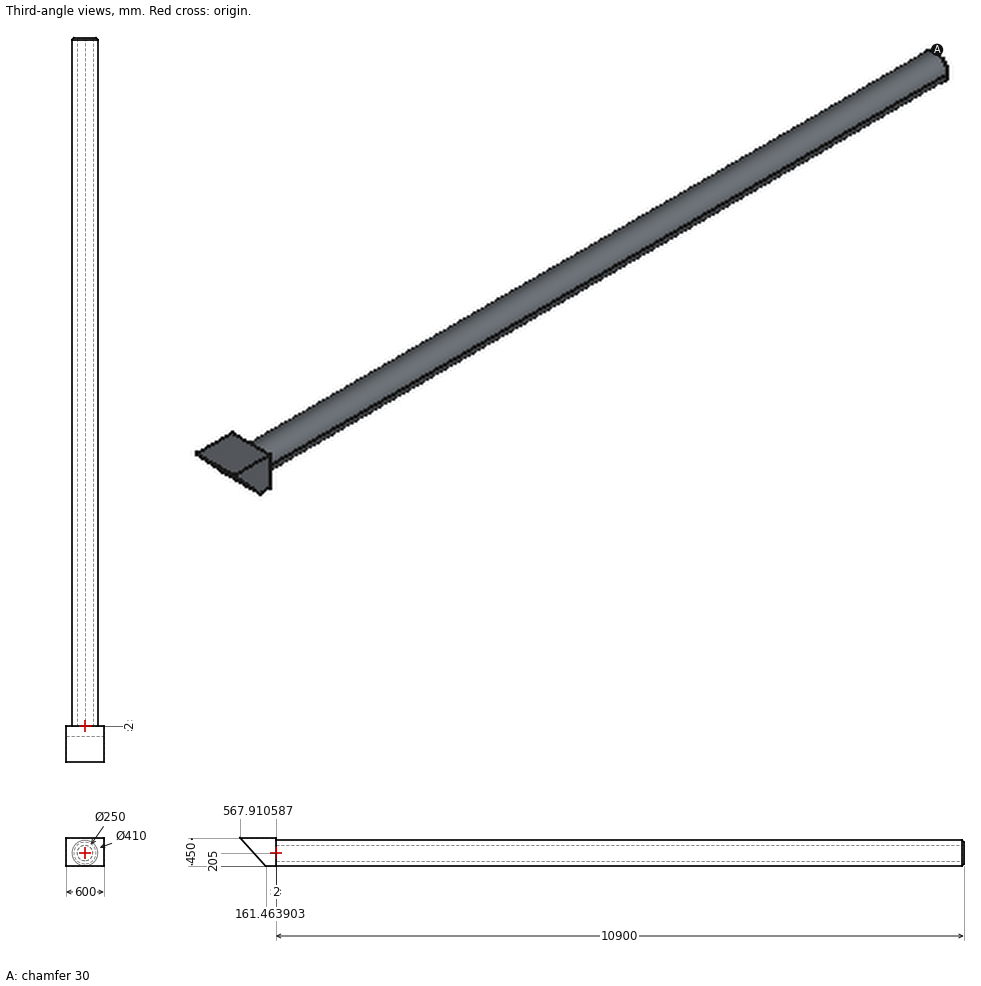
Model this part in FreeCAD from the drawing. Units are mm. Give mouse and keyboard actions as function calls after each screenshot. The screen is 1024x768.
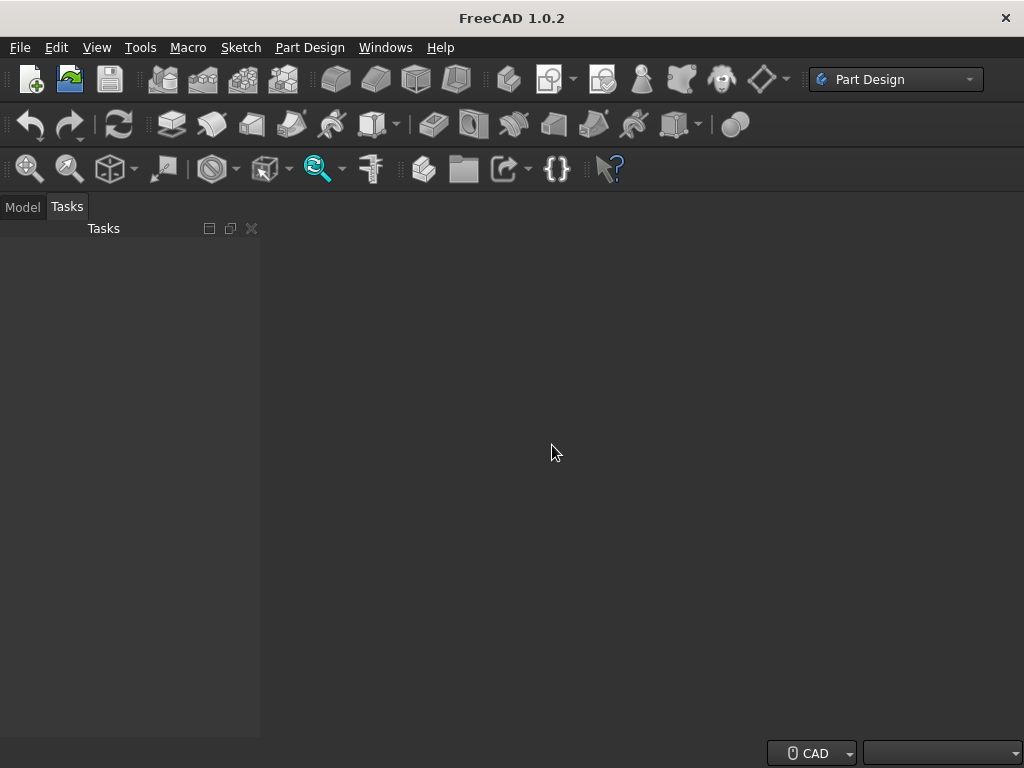
click(30, 80)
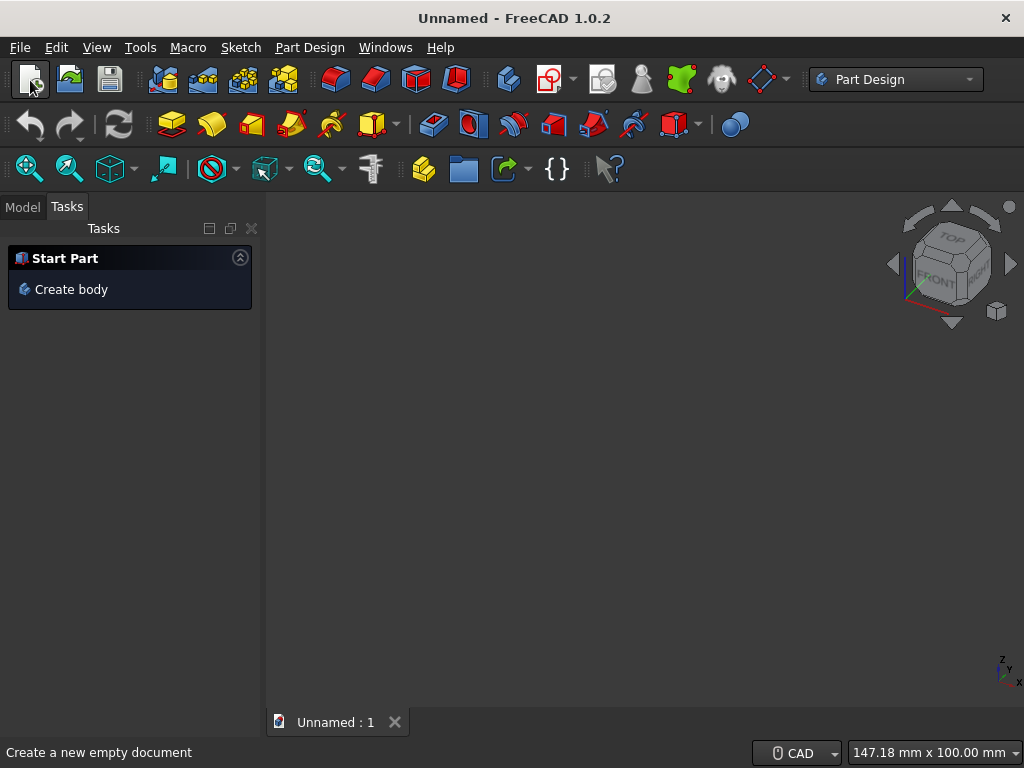
click(550, 80)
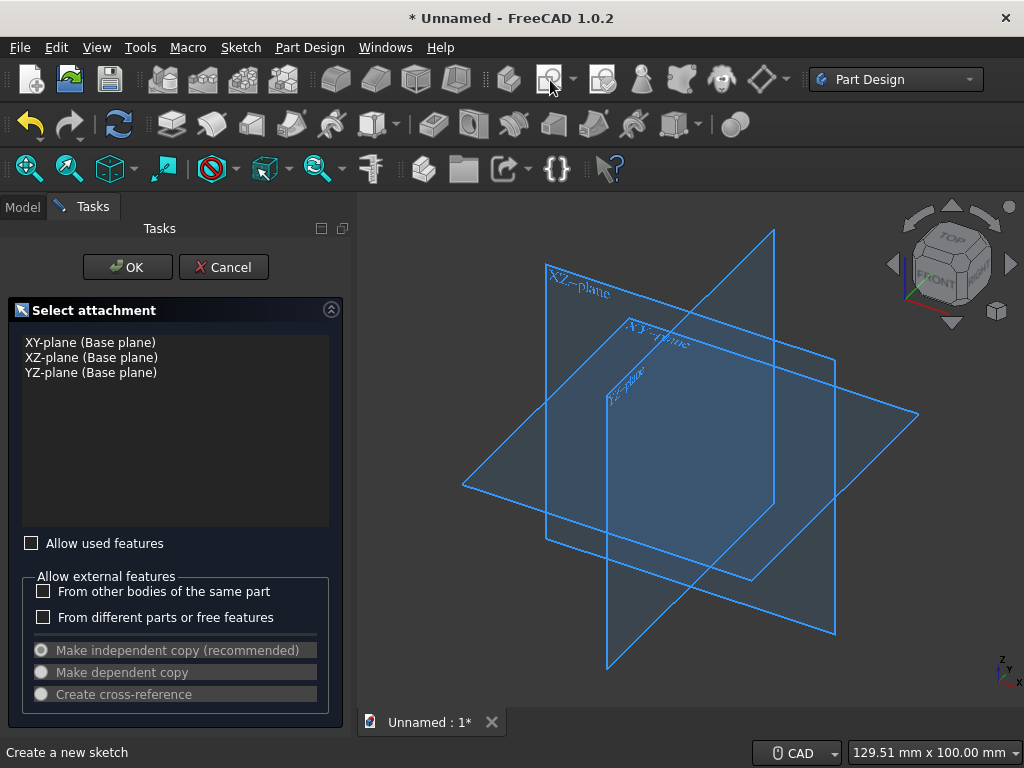
click(82, 358)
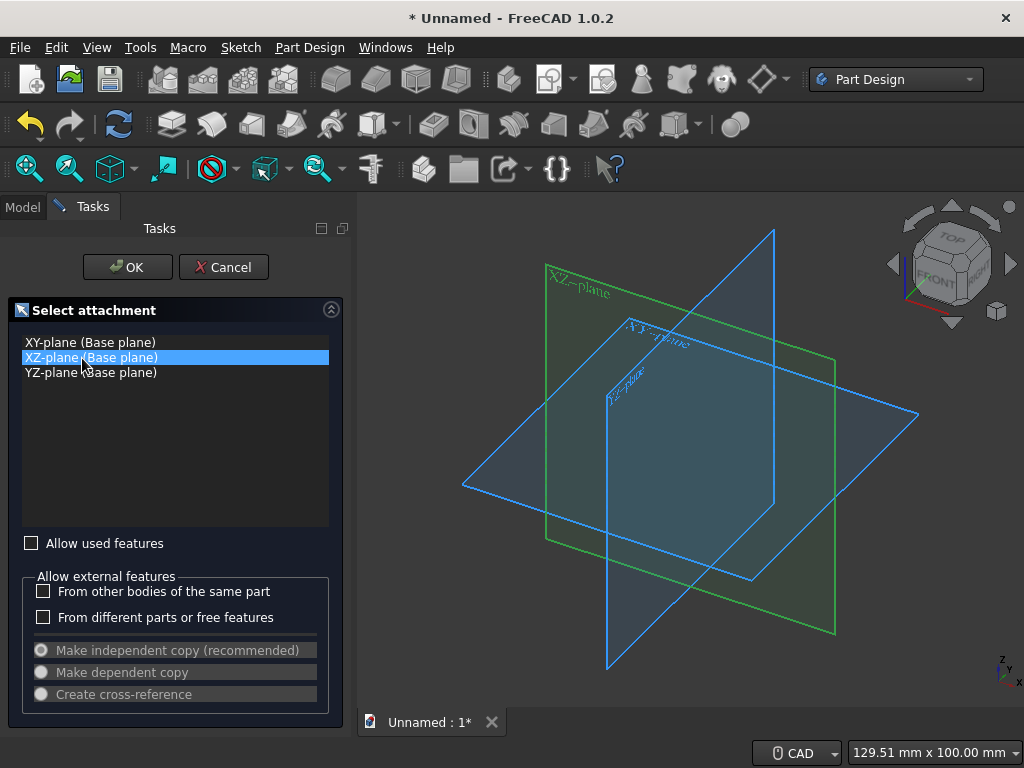
click(128, 267)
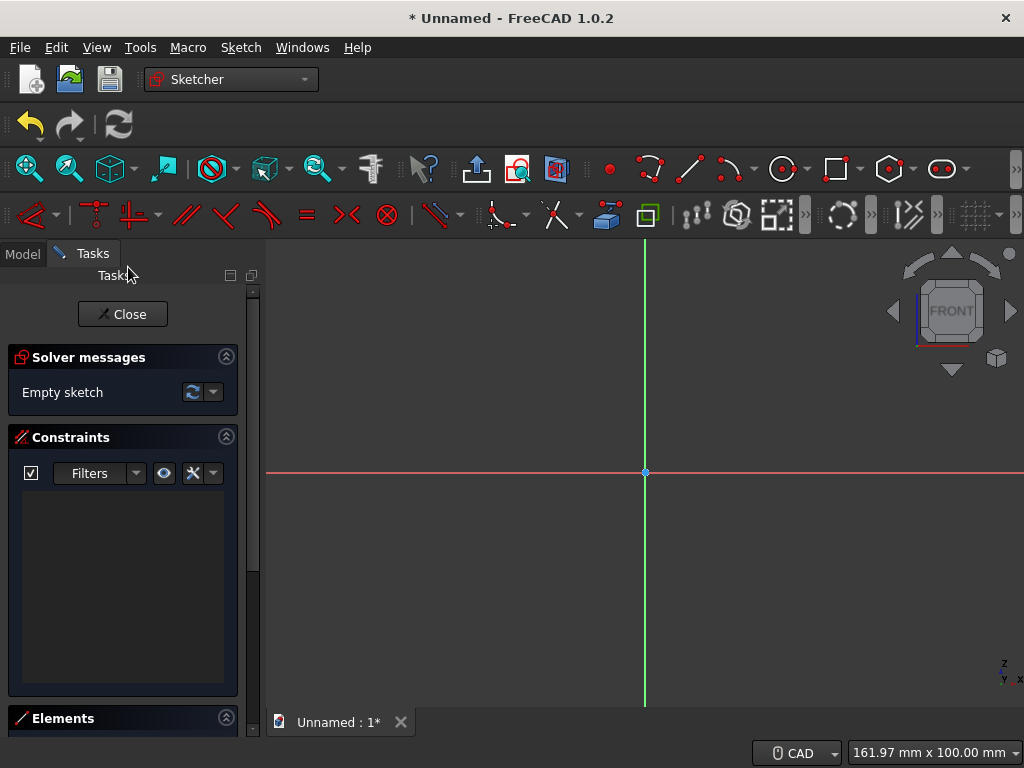
scroll(563, 473, down, 9)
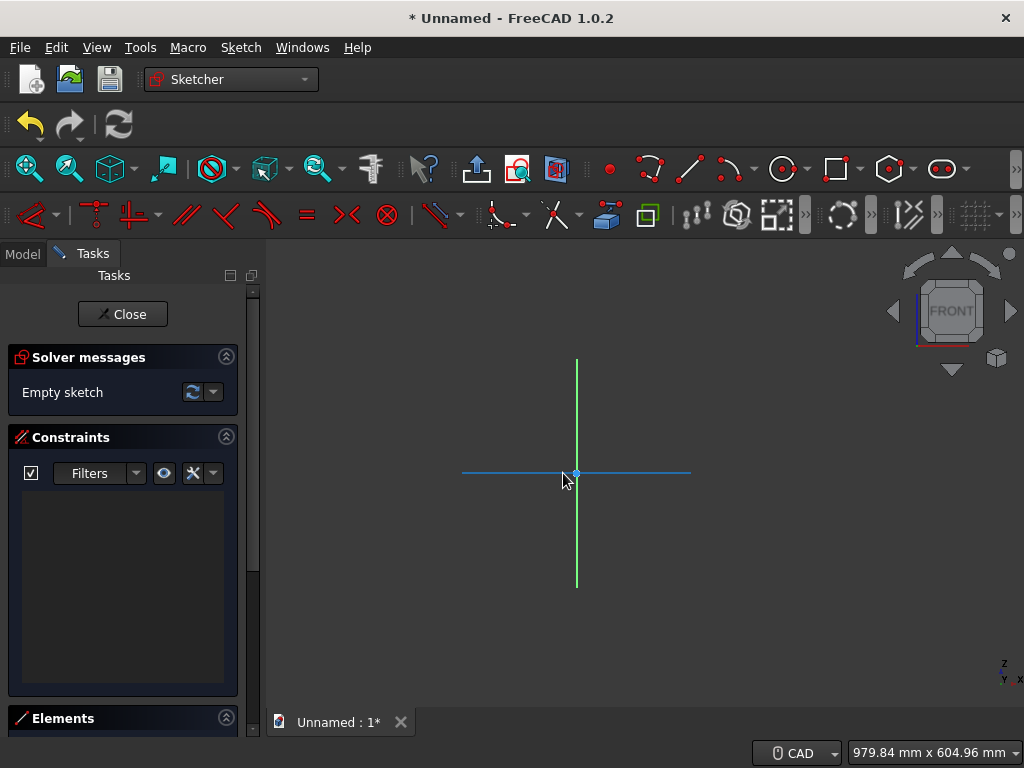
click(784, 170)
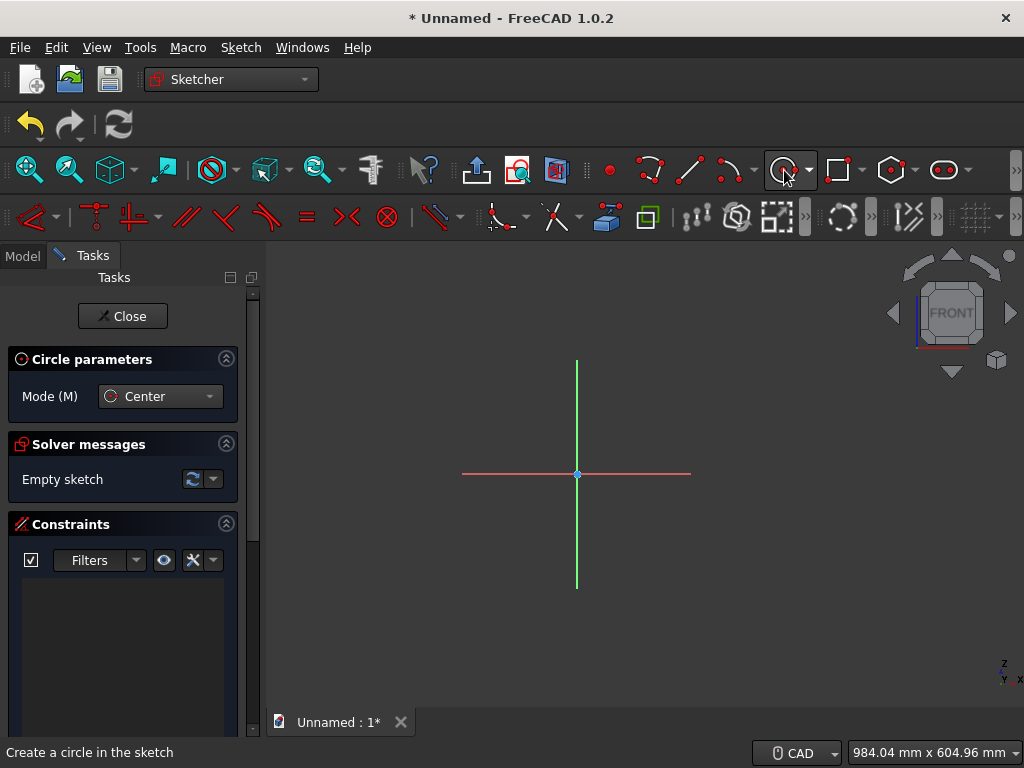
click(577, 474)
move(689, 363)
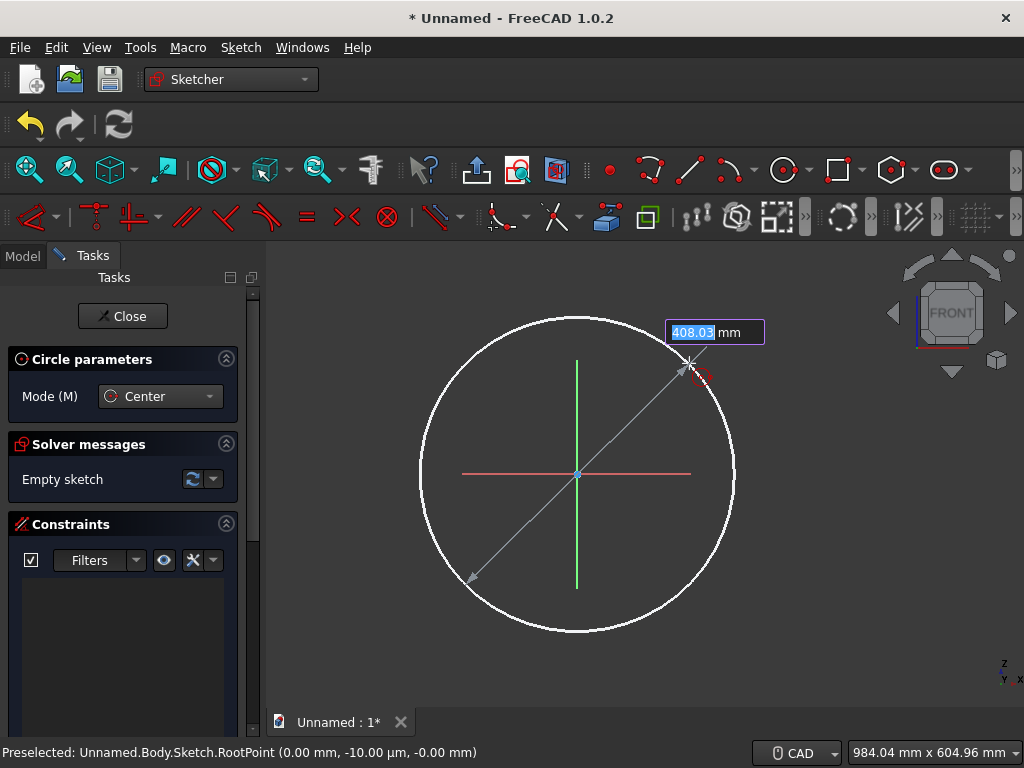
text(410)
key(Return)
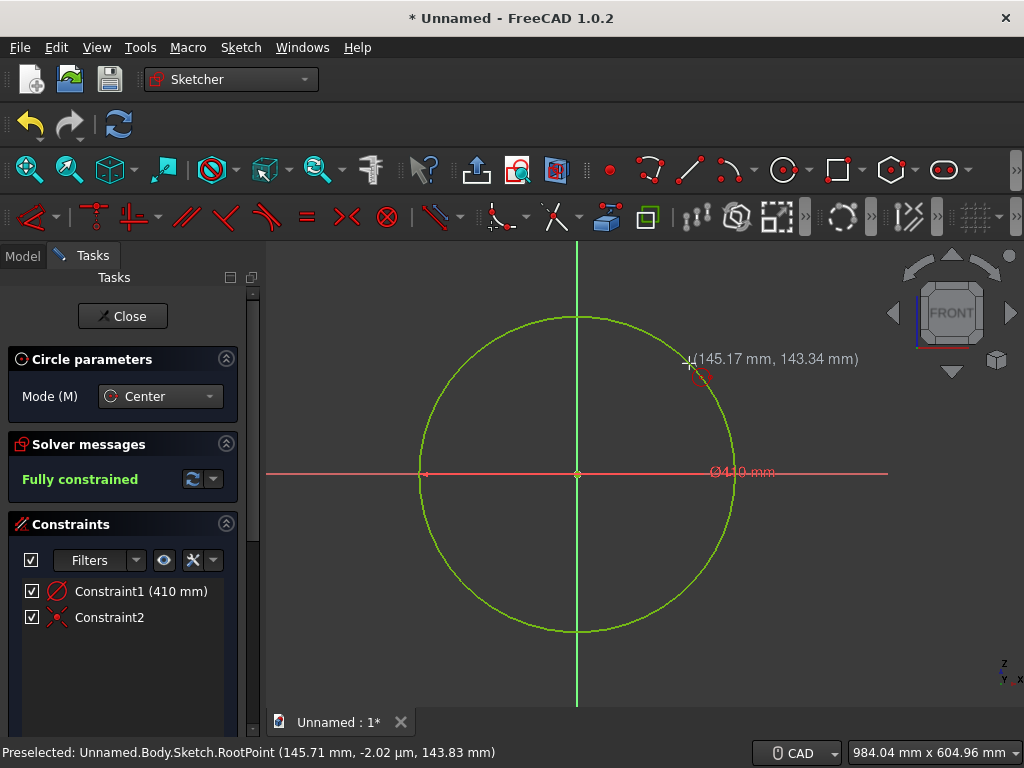
click(577, 474)
move(645, 406)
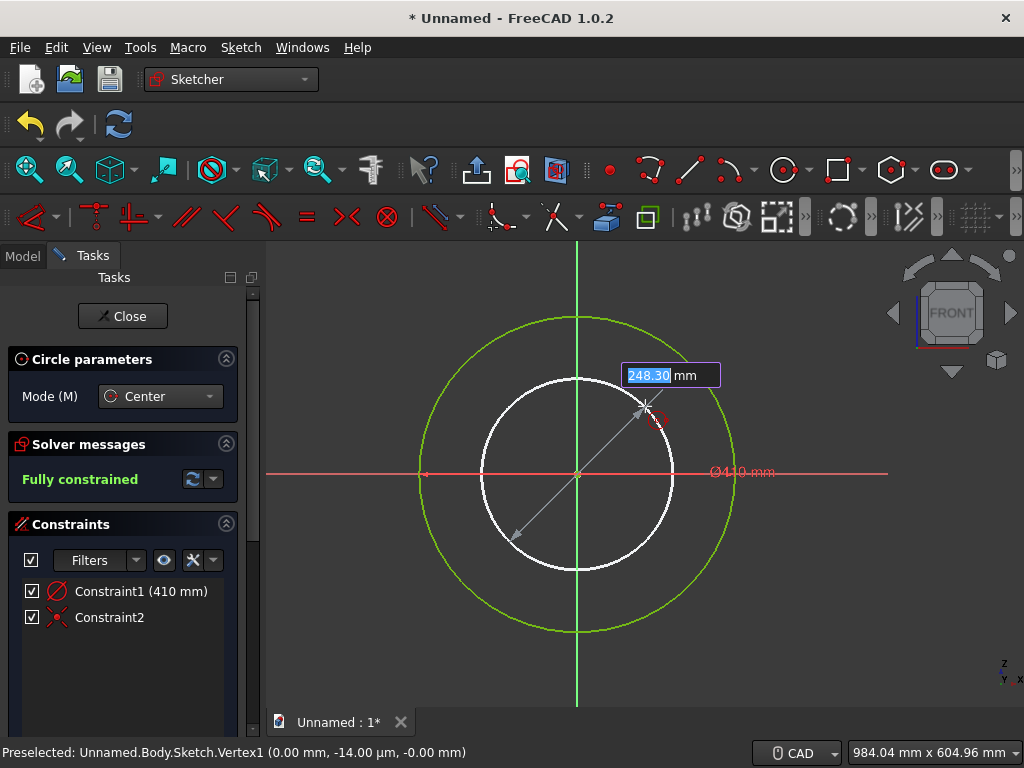
text(250)
key(Return)
key(Escape)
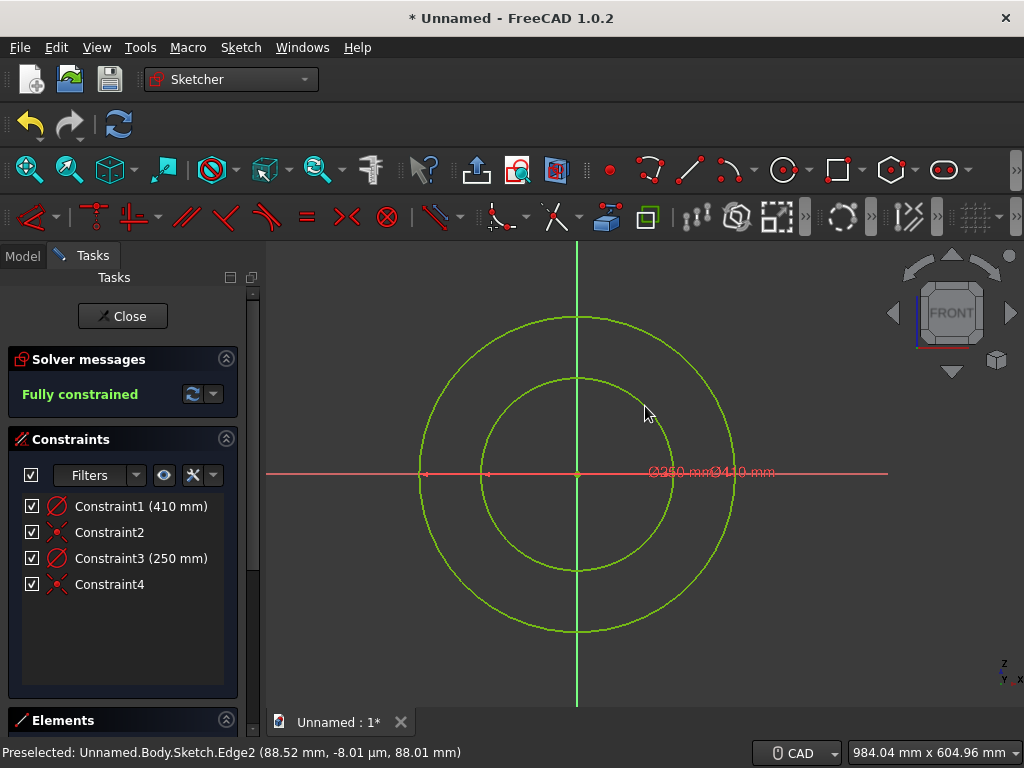
click(123, 316)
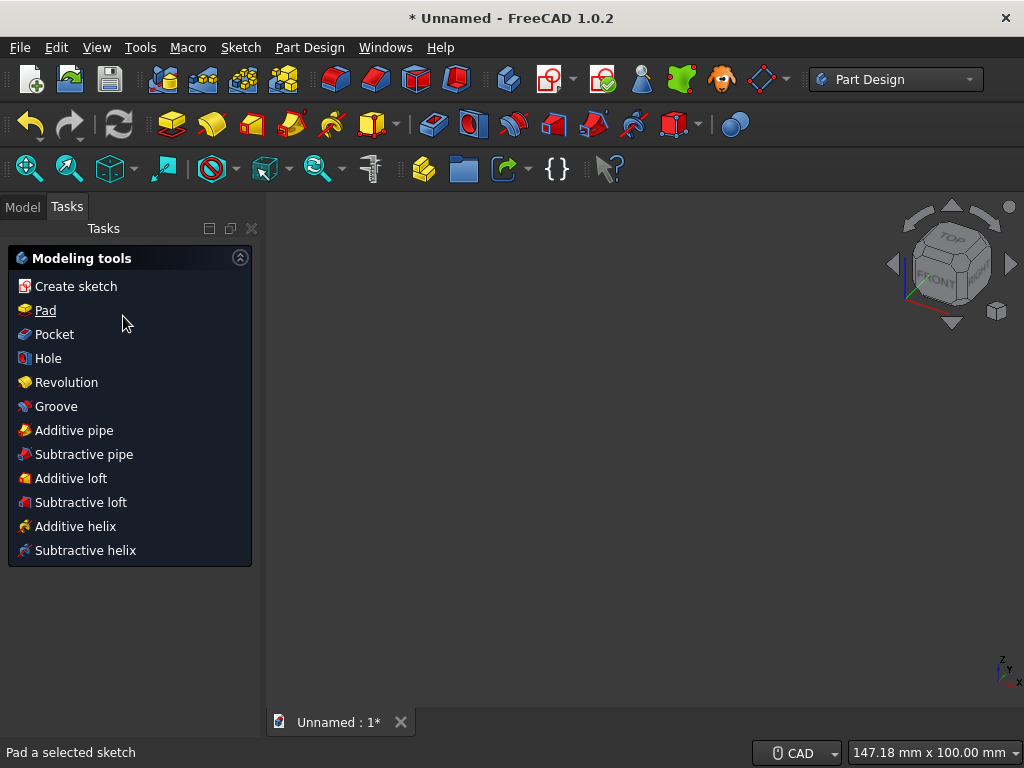
click(172, 124)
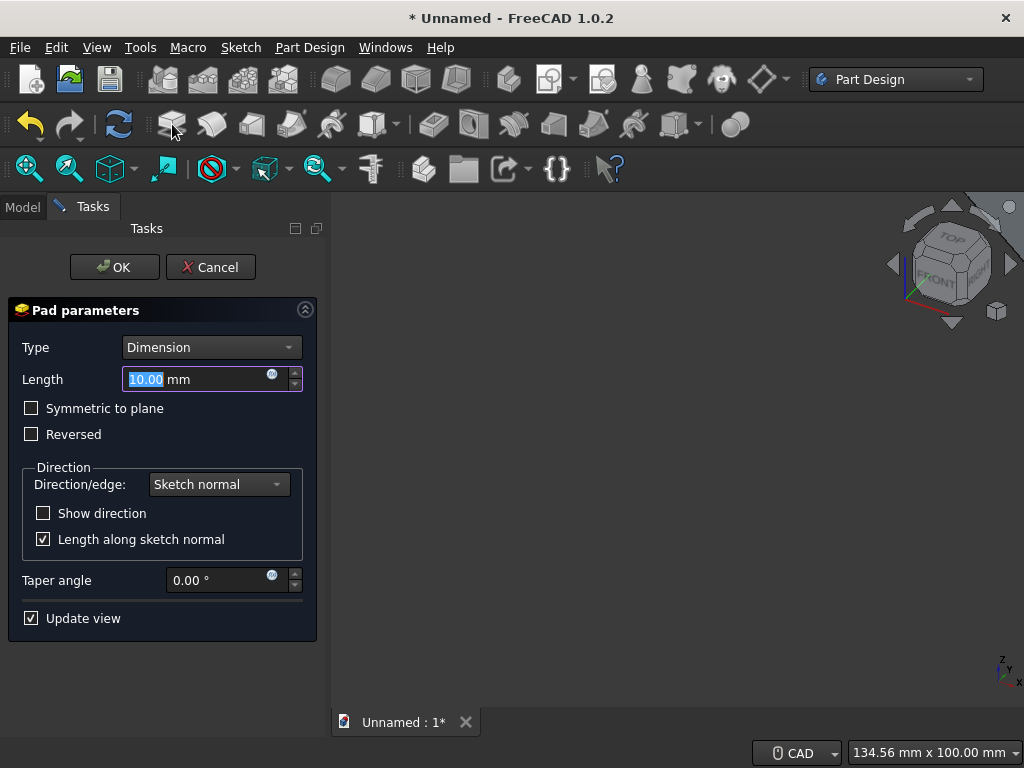
text(10900)
key(Tab)